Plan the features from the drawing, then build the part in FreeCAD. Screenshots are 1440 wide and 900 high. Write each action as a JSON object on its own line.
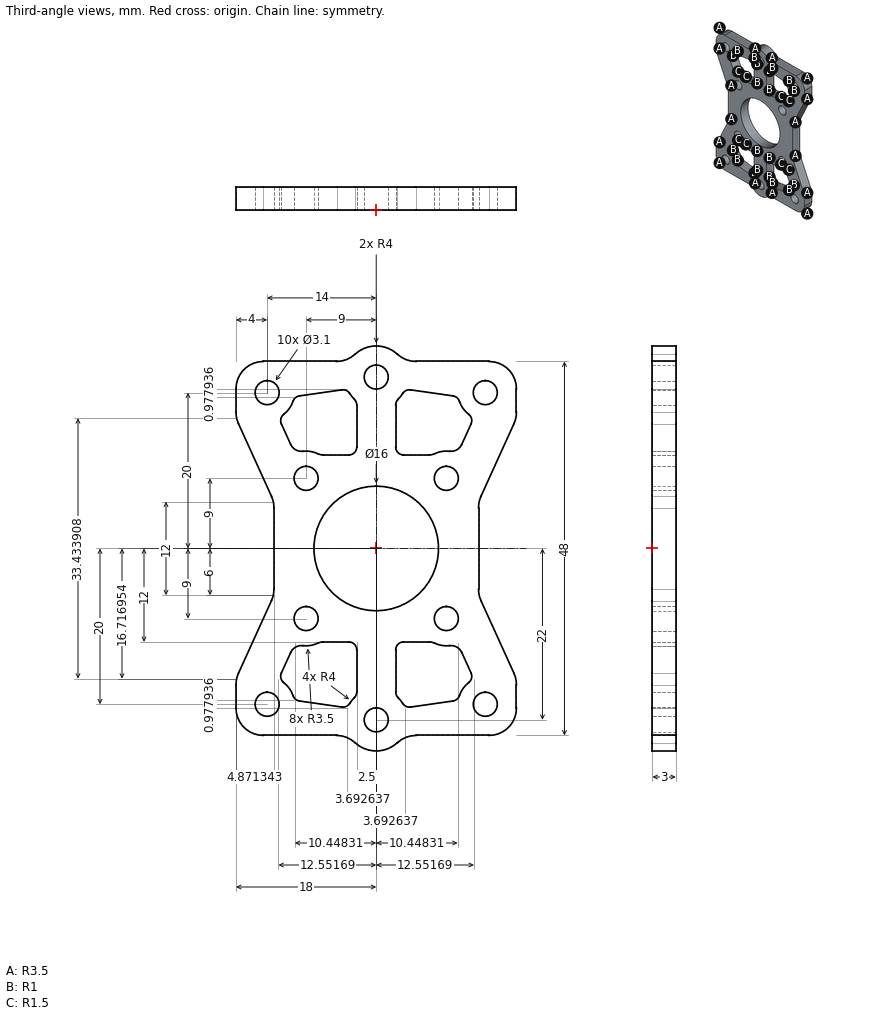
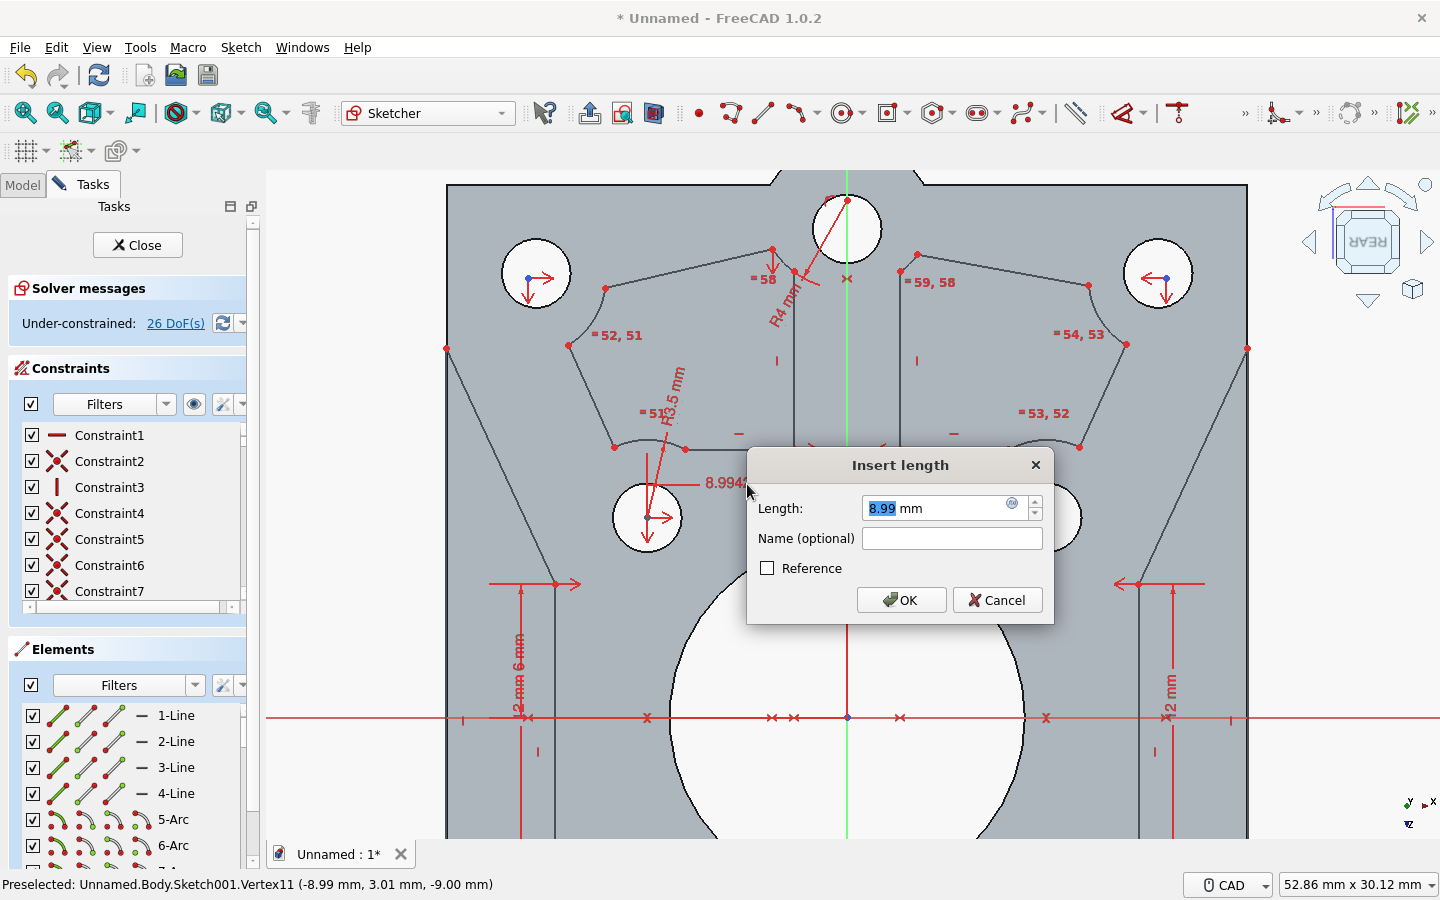
{"action": "type", "text": "9"}
{"action": "key", "text": "Return"}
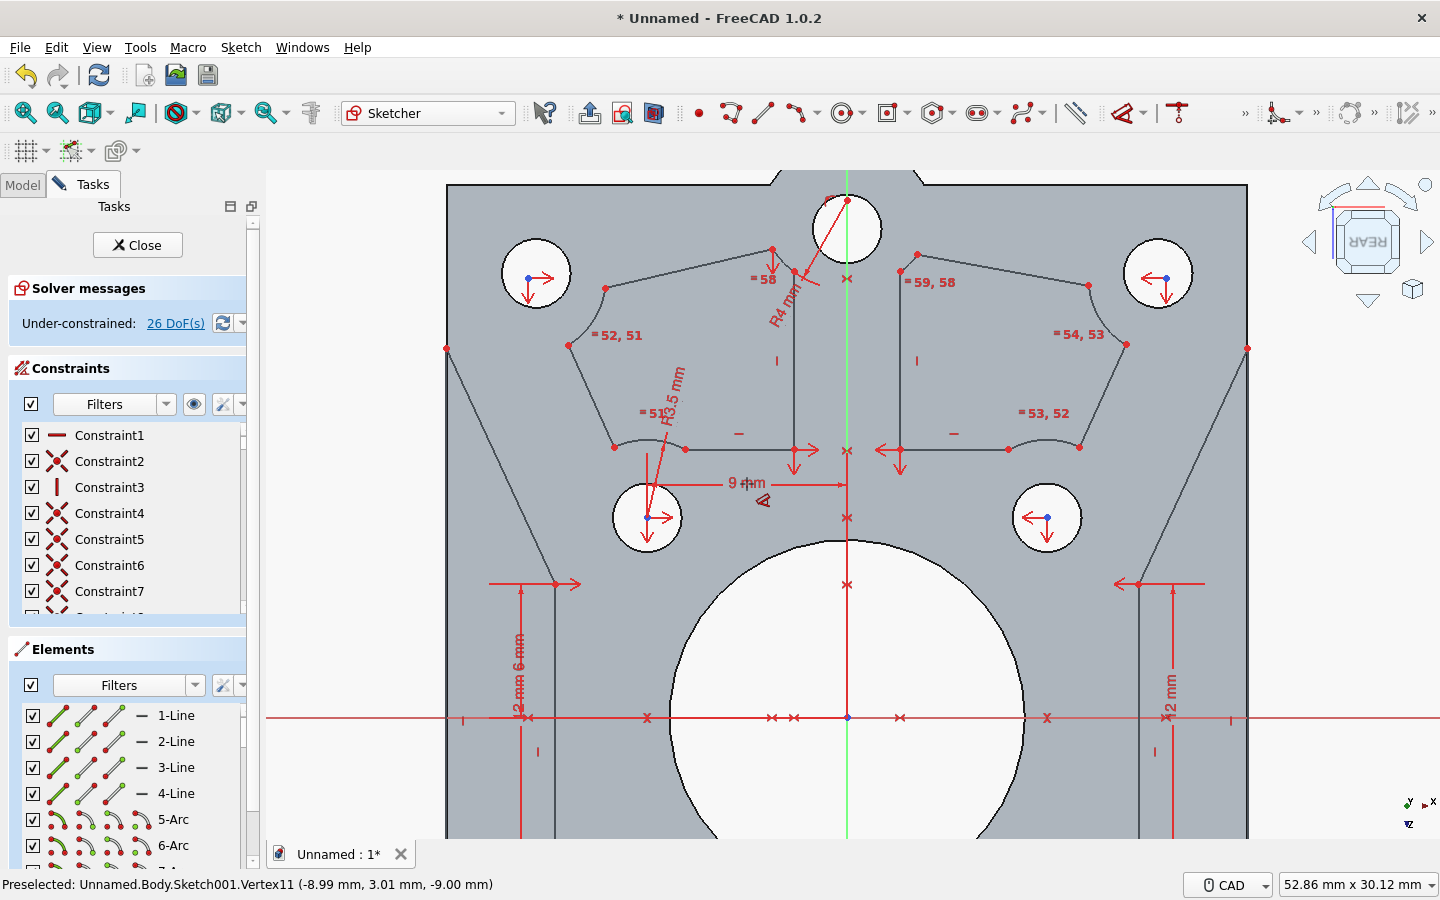
{"action": "left_click", "coordinate": [647, 518]}
{"action": "left_click", "coordinate": [613, 618]}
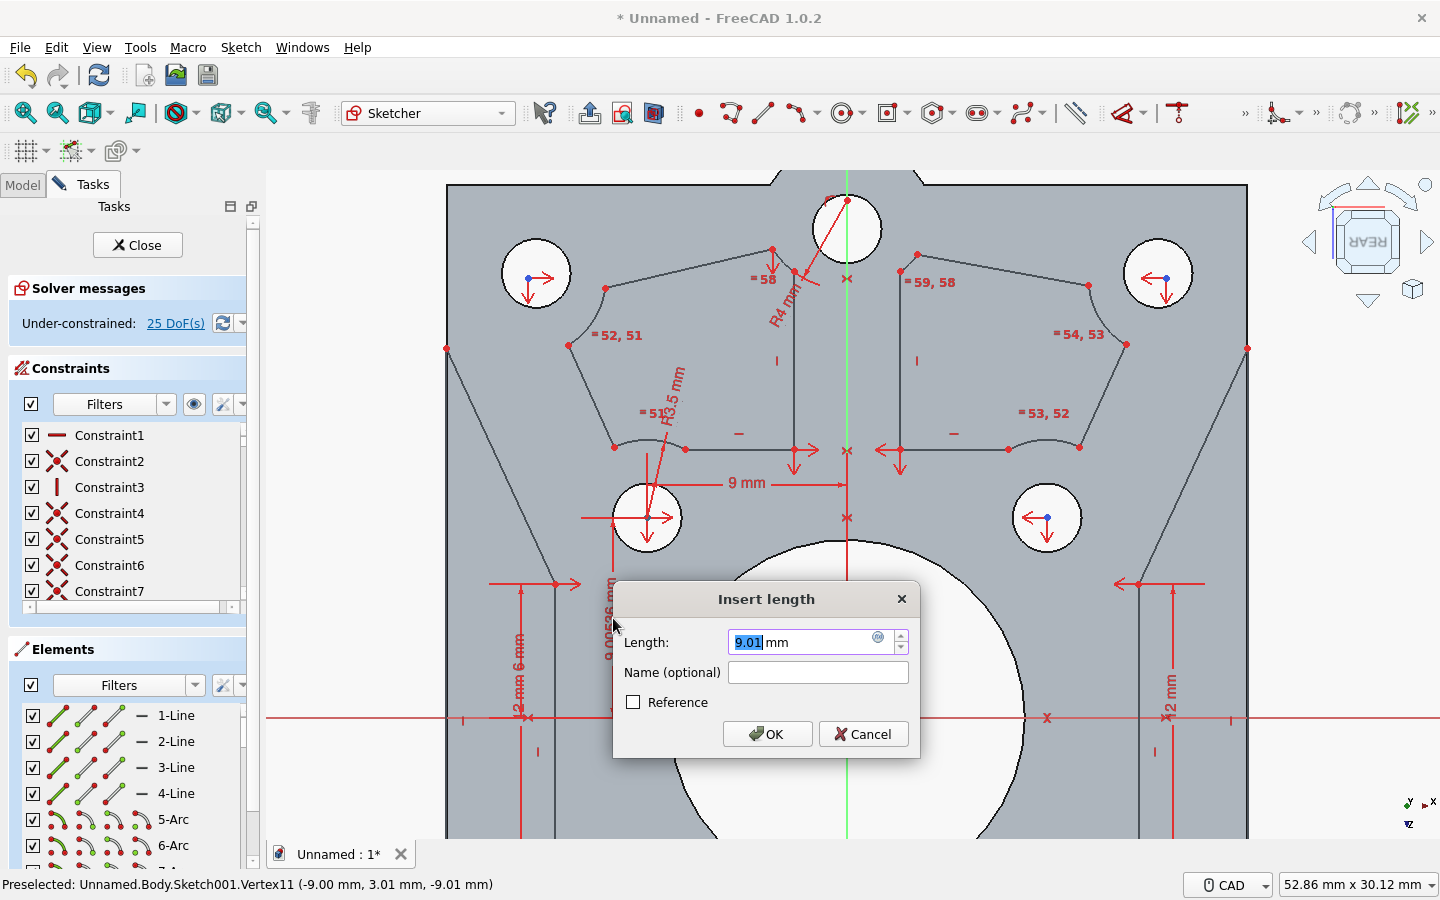
{"action": "type", "text": "9"}
{"action": "key", "text": "Return"}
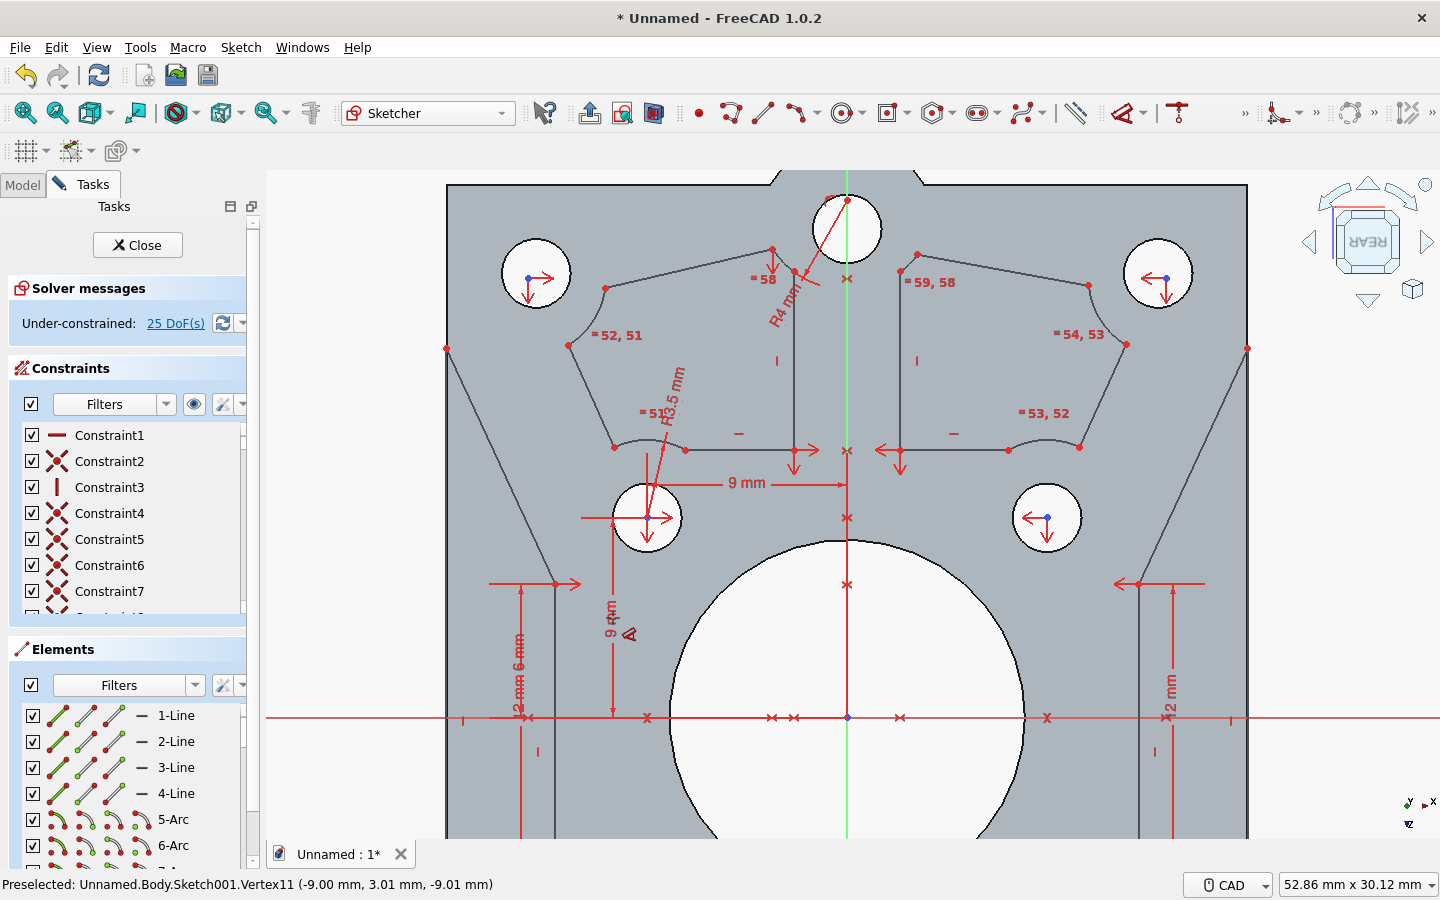
{"action": "left_click", "coordinate": [686, 450]}
{"action": "left_click", "coordinate": [652, 584]}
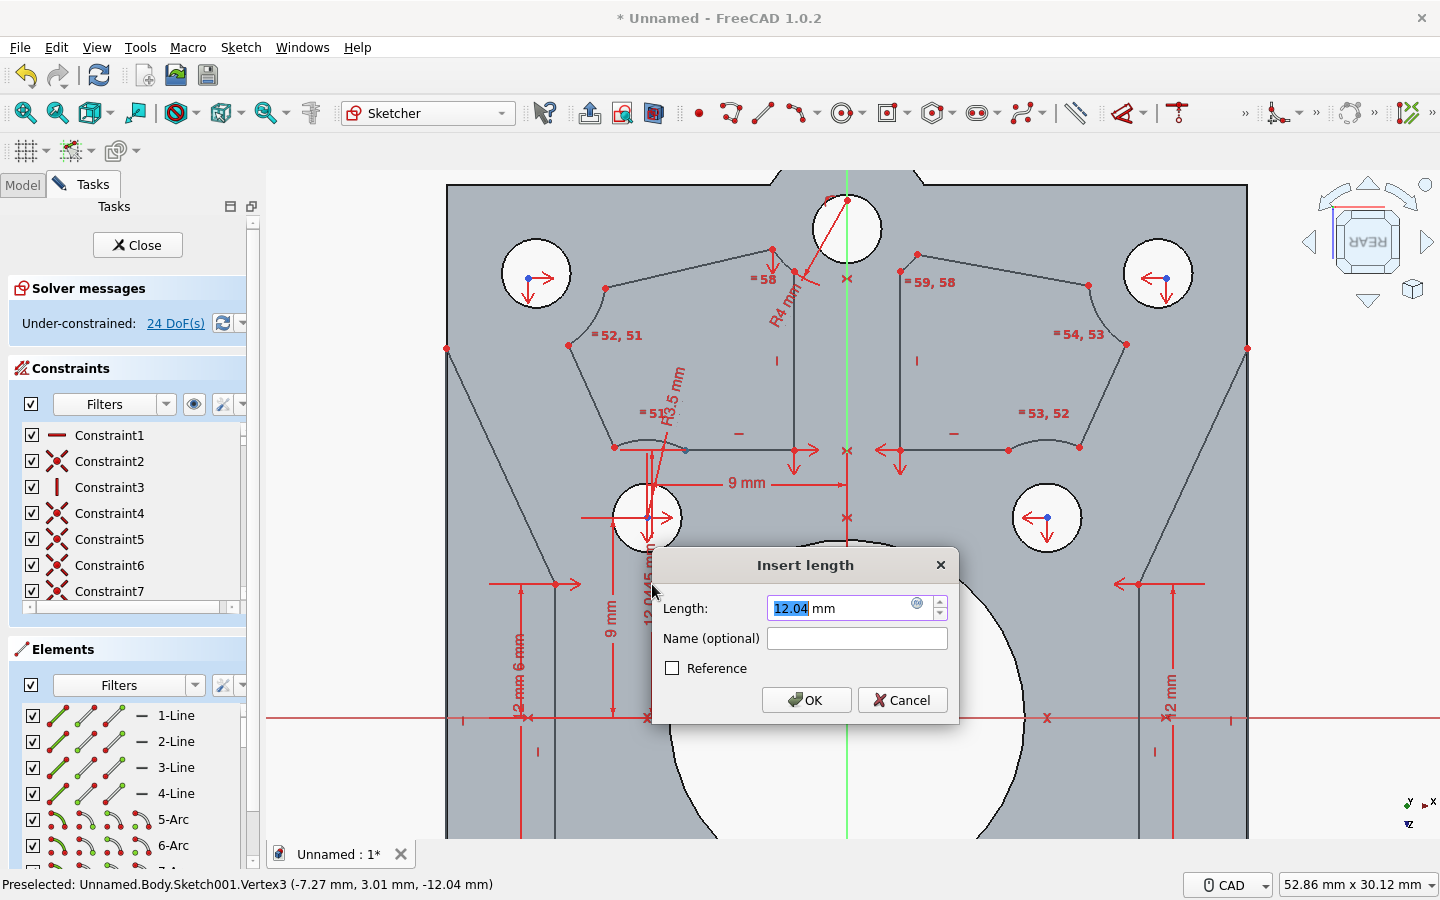
{"action": "type", "text": "12"}
{"action": "key", "text": "Return"}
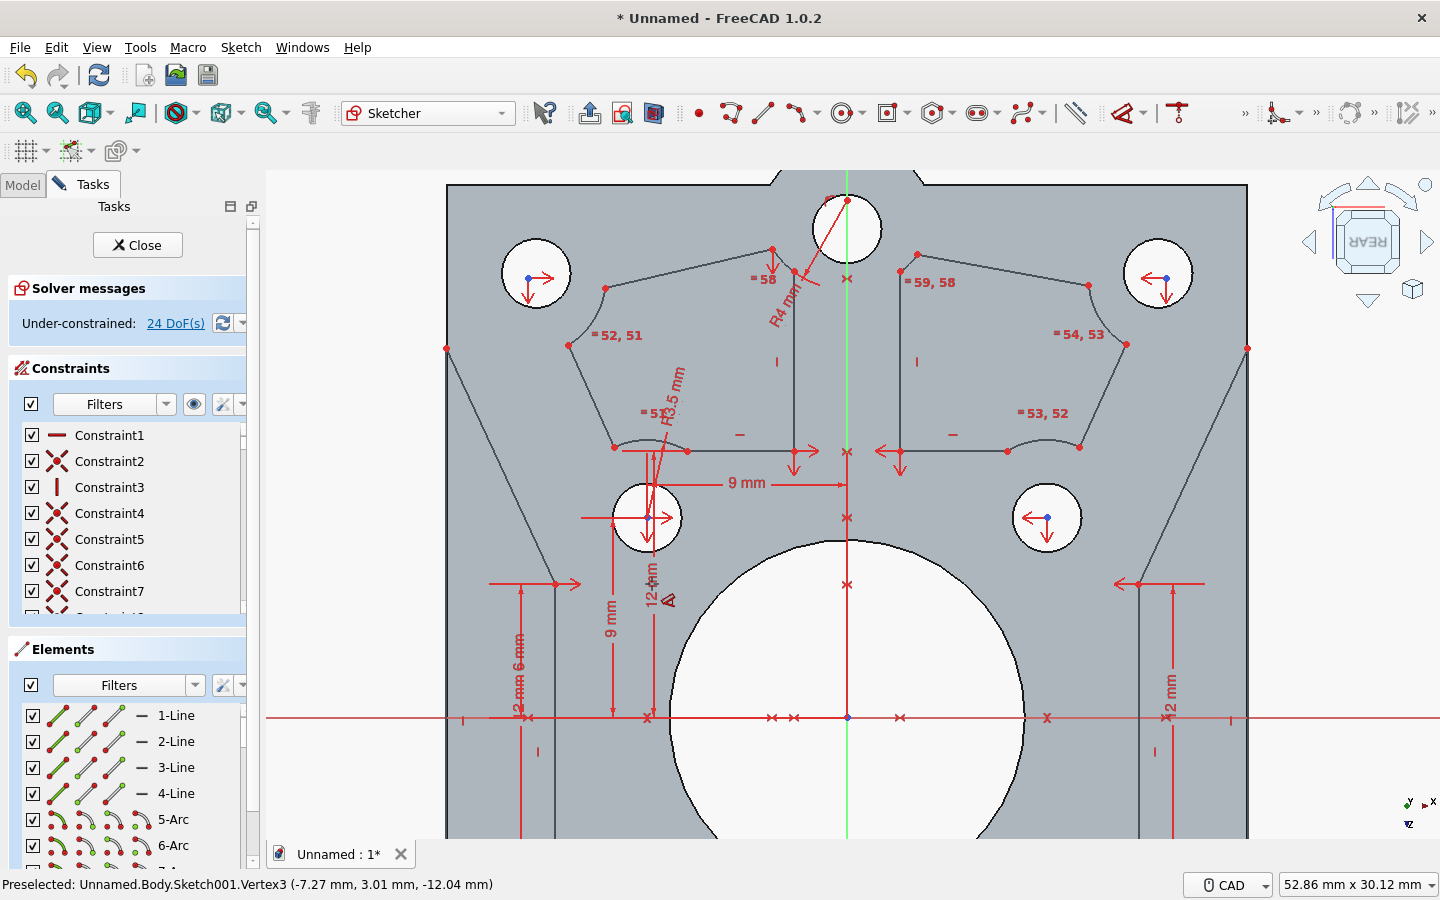
{"action": "left_click", "coordinate": [446, 349]}
{"action": "left_click", "coordinate": [647, 315]}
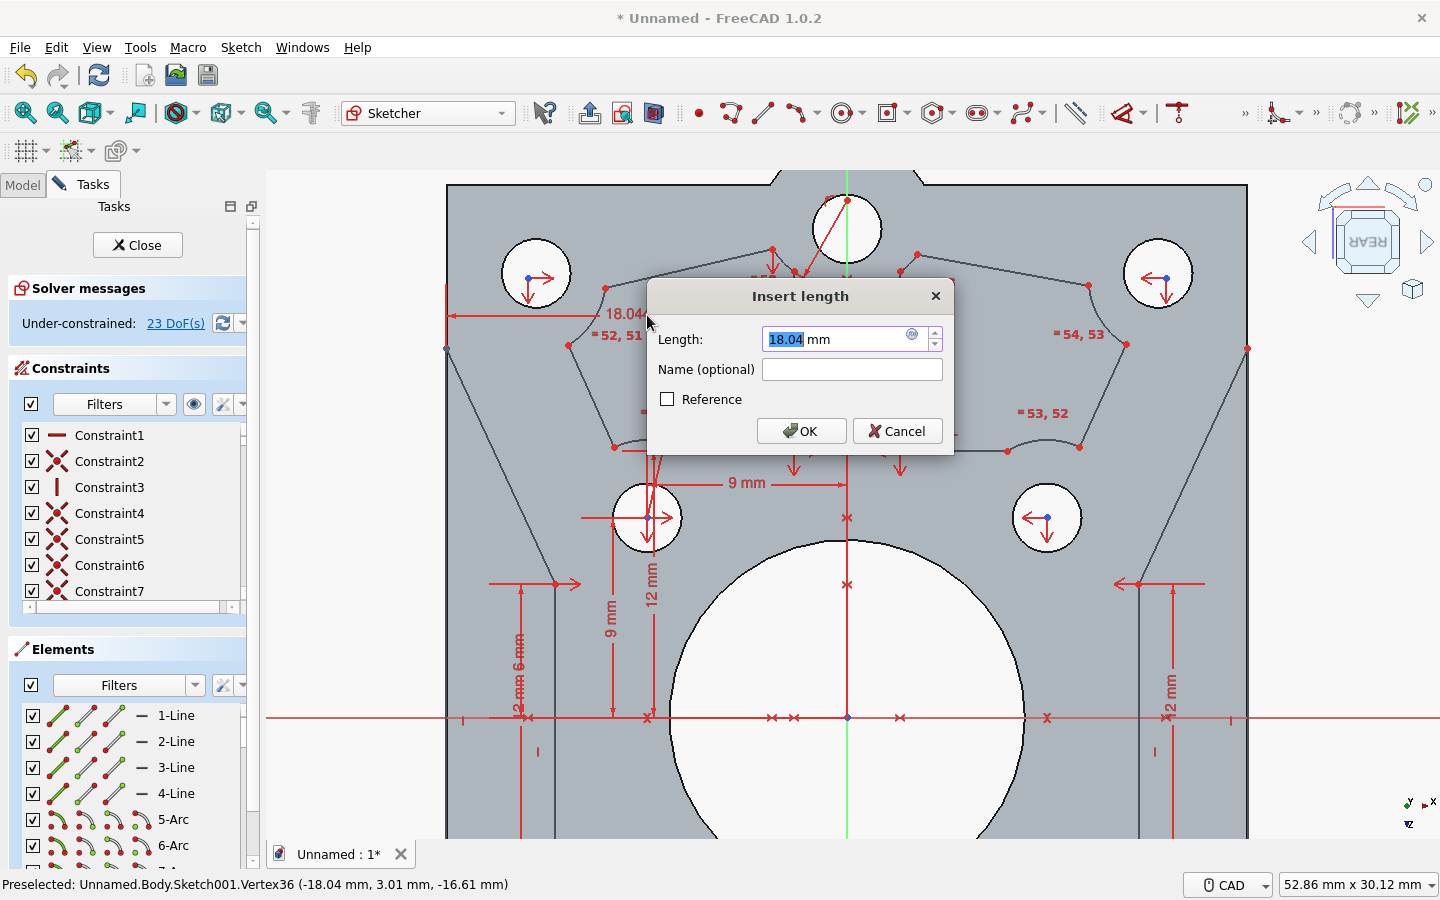
{"action": "type", "text": "18"}
{"action": "key", "text": "Return"}